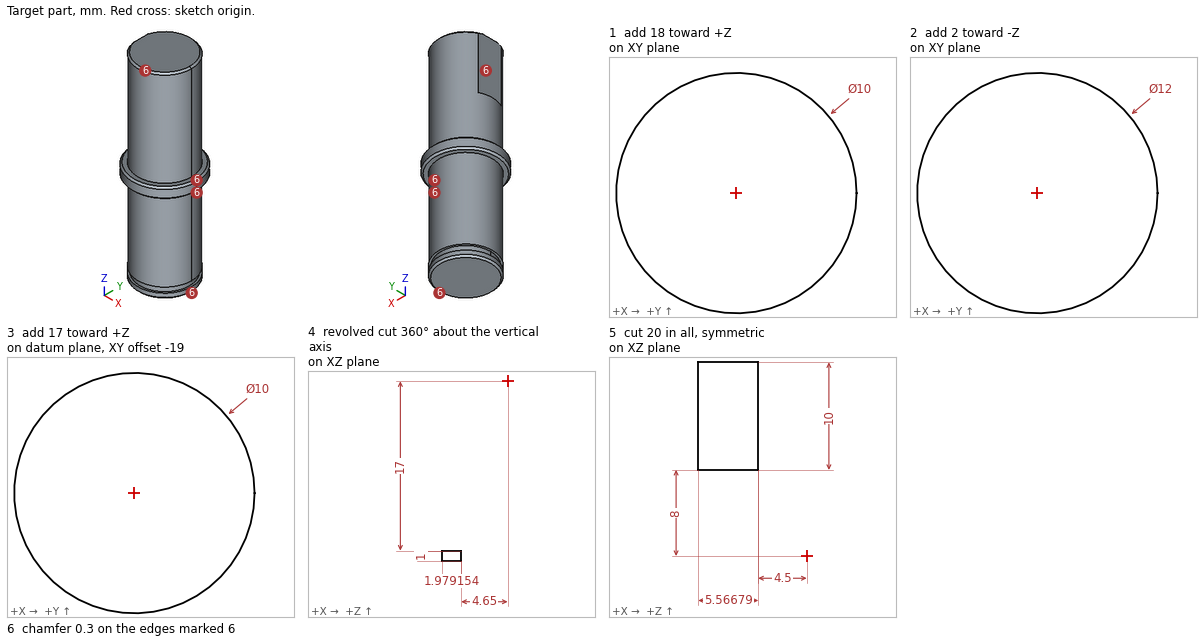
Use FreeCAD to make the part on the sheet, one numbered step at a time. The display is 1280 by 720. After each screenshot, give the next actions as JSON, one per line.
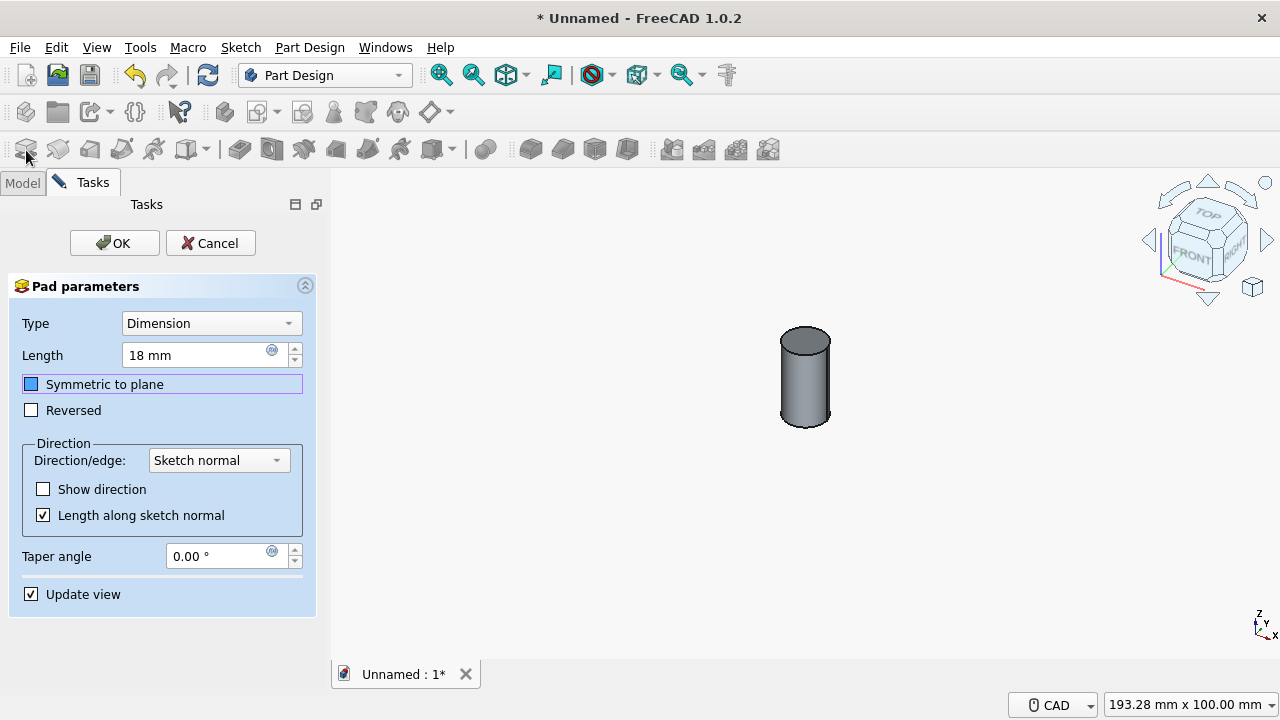
{"action": "left_click", "coordinate": [115, 243]}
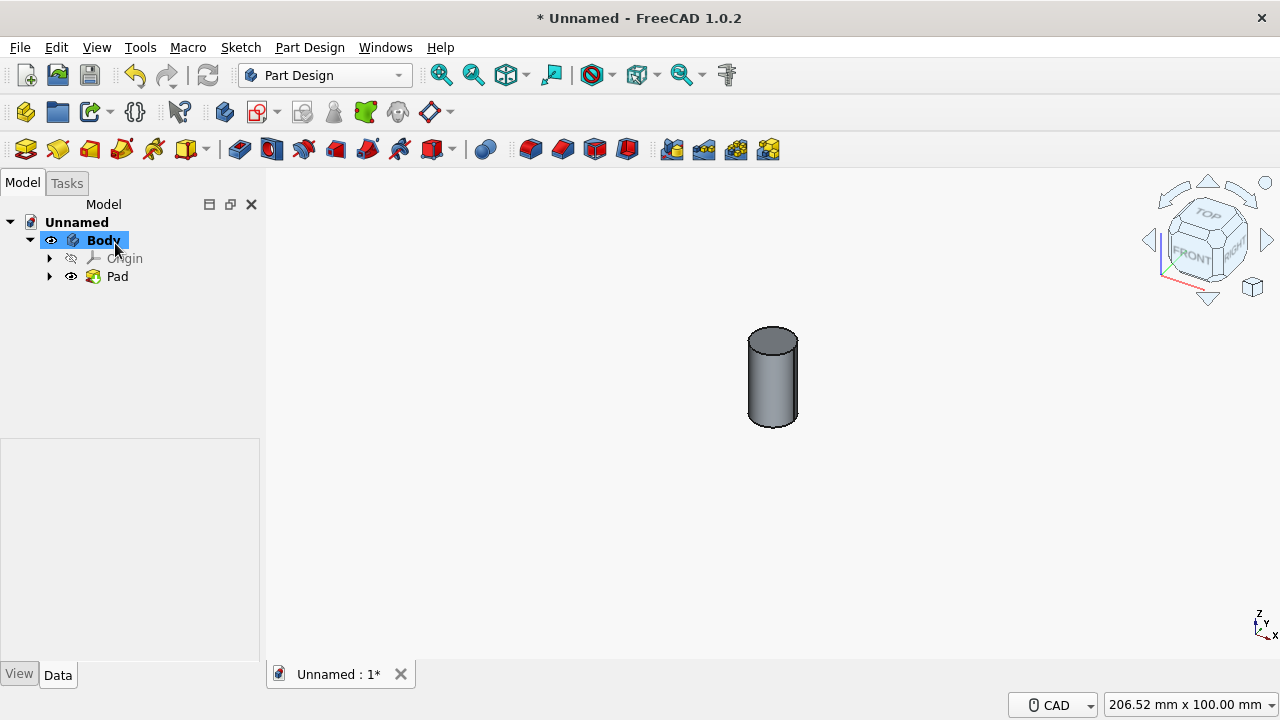
{"action": "left_click", "coordinate": [442, 76]}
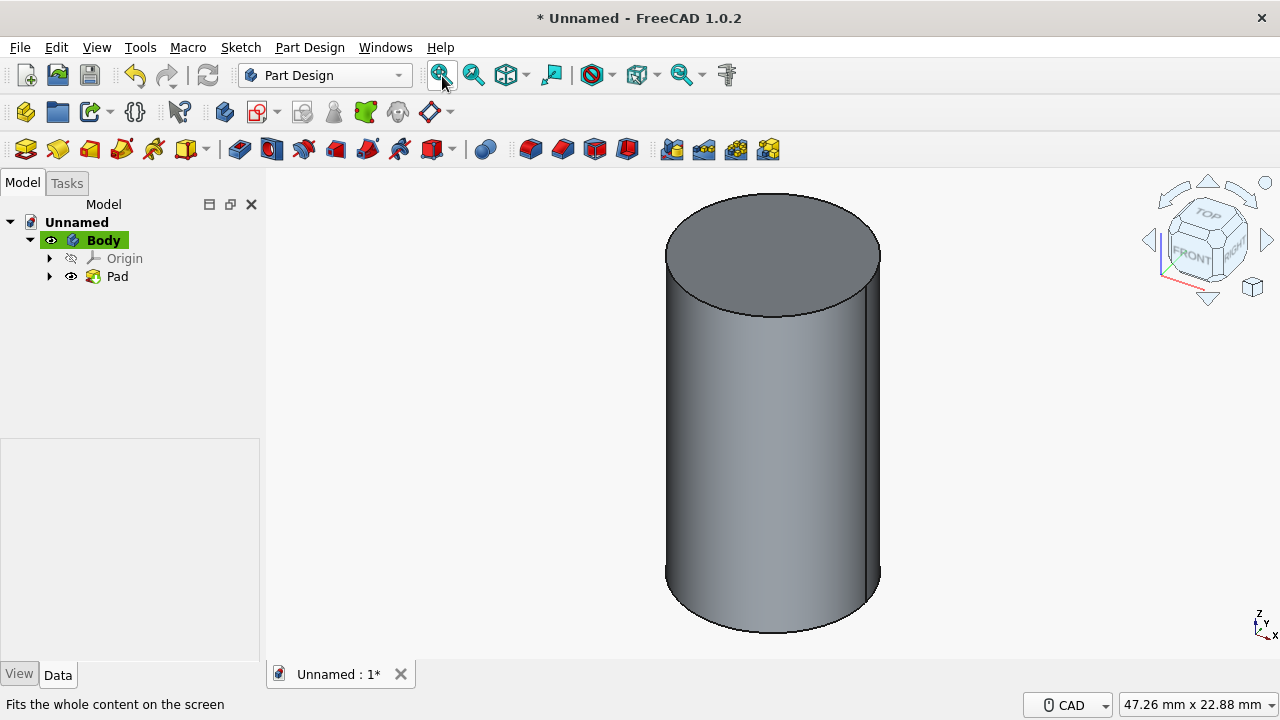
{"action": "left_click", "coordinate": [258, 112]}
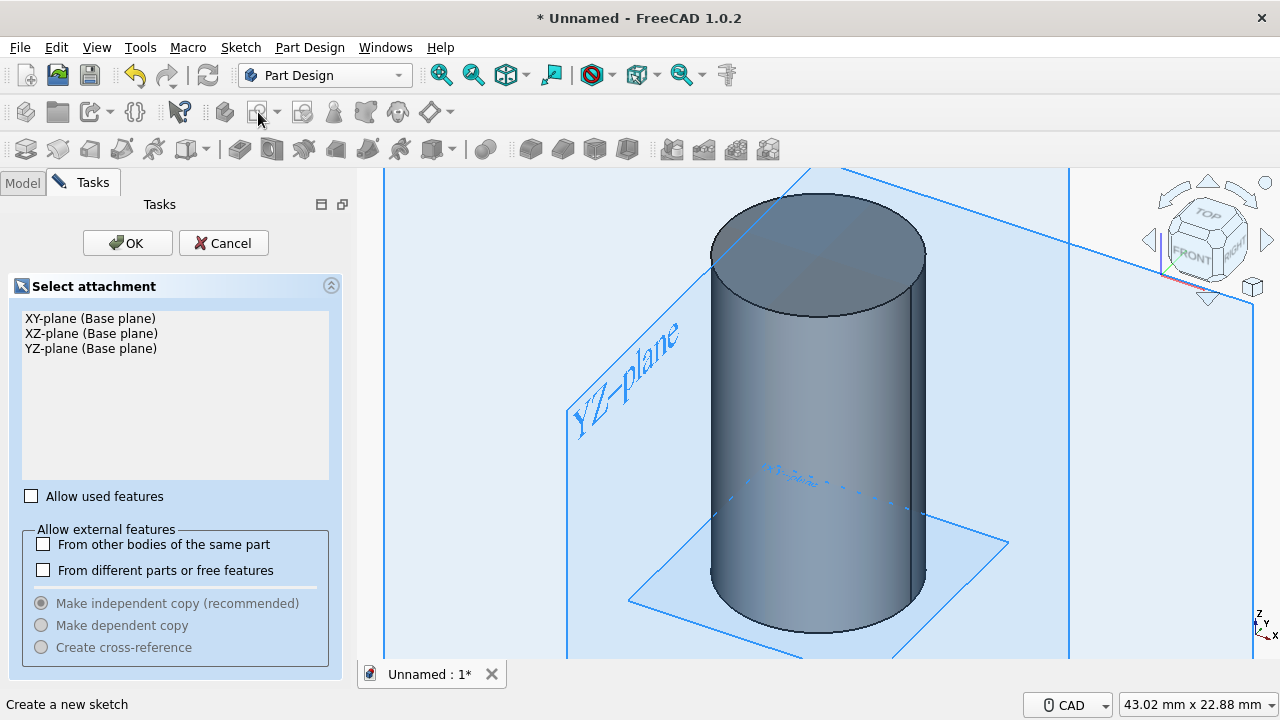
{"action": "left_click", "coordinate": [82, 318]}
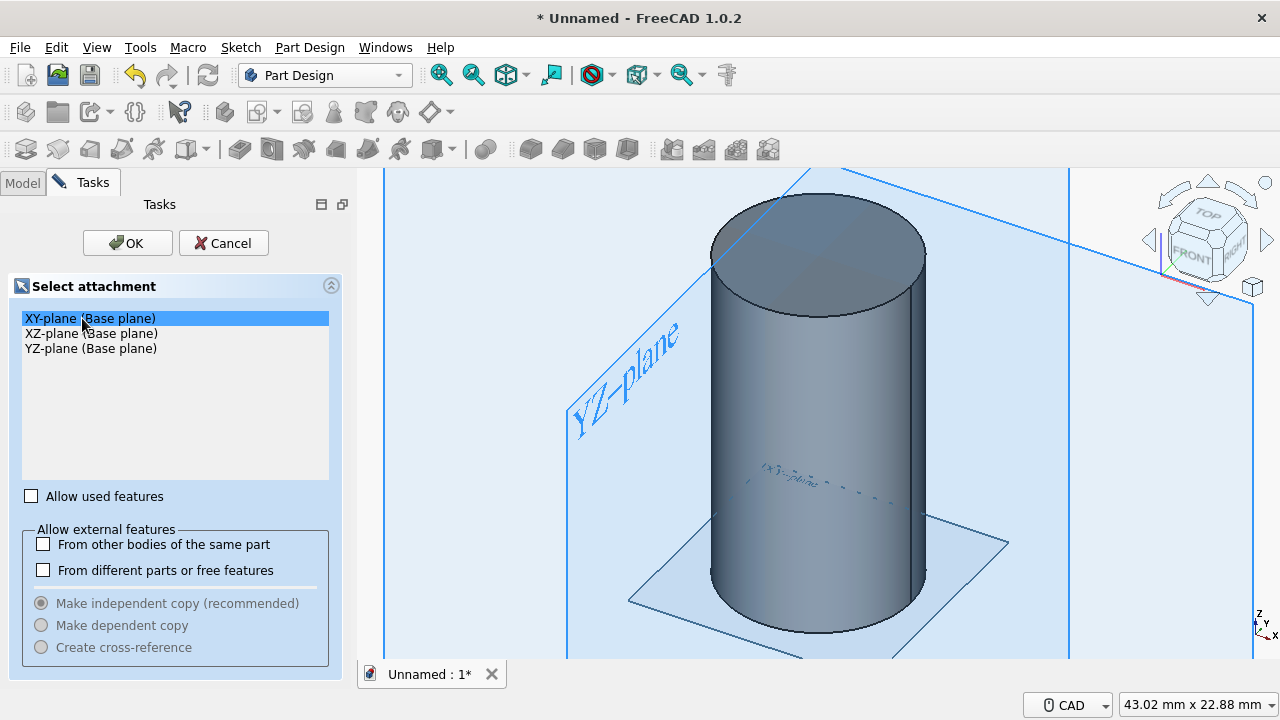
{"action": "left_click", "coordinate": [128, 243]}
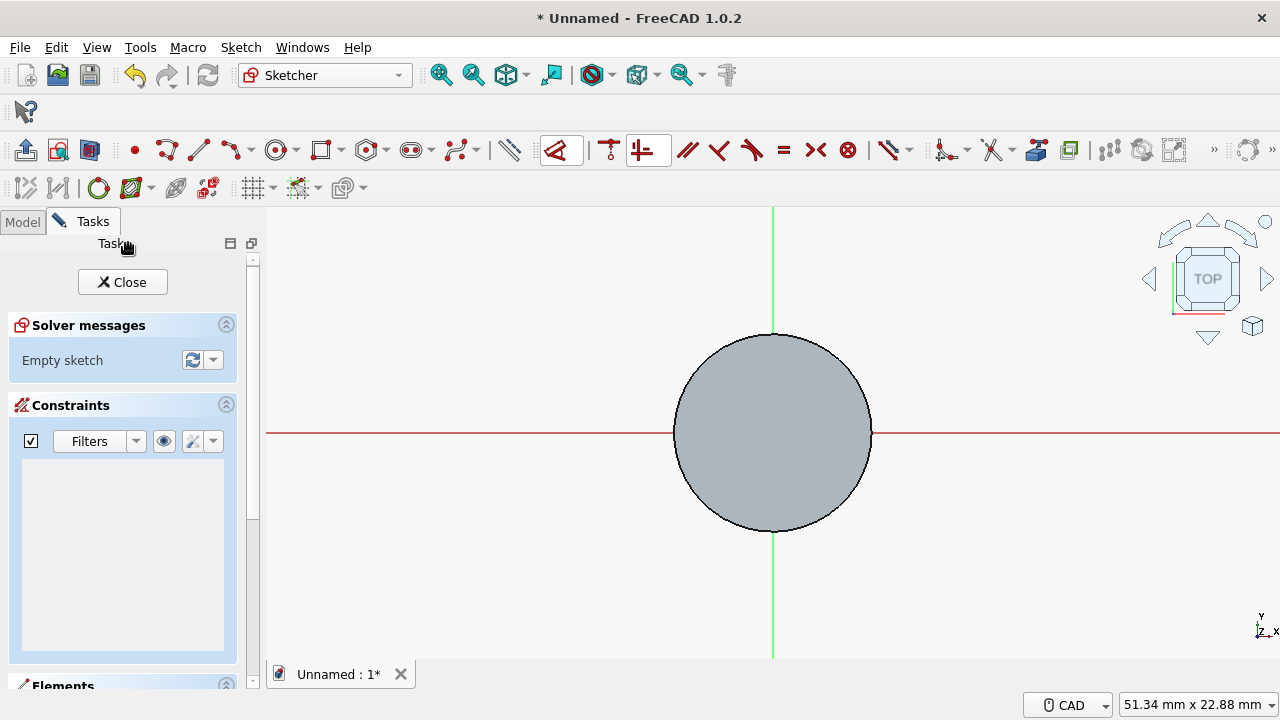
{"action": "left_click", "coordinate": [90, 150]}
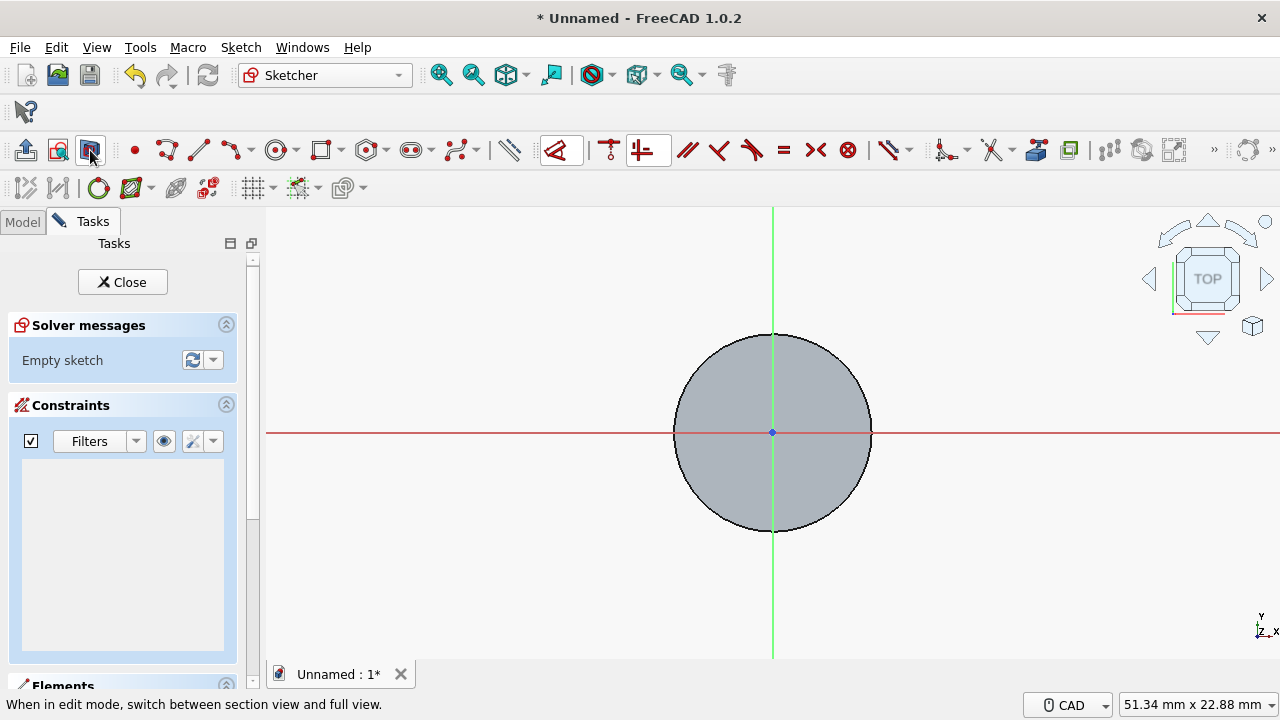
{"action": "left_click", "coordinate": [276, 150]}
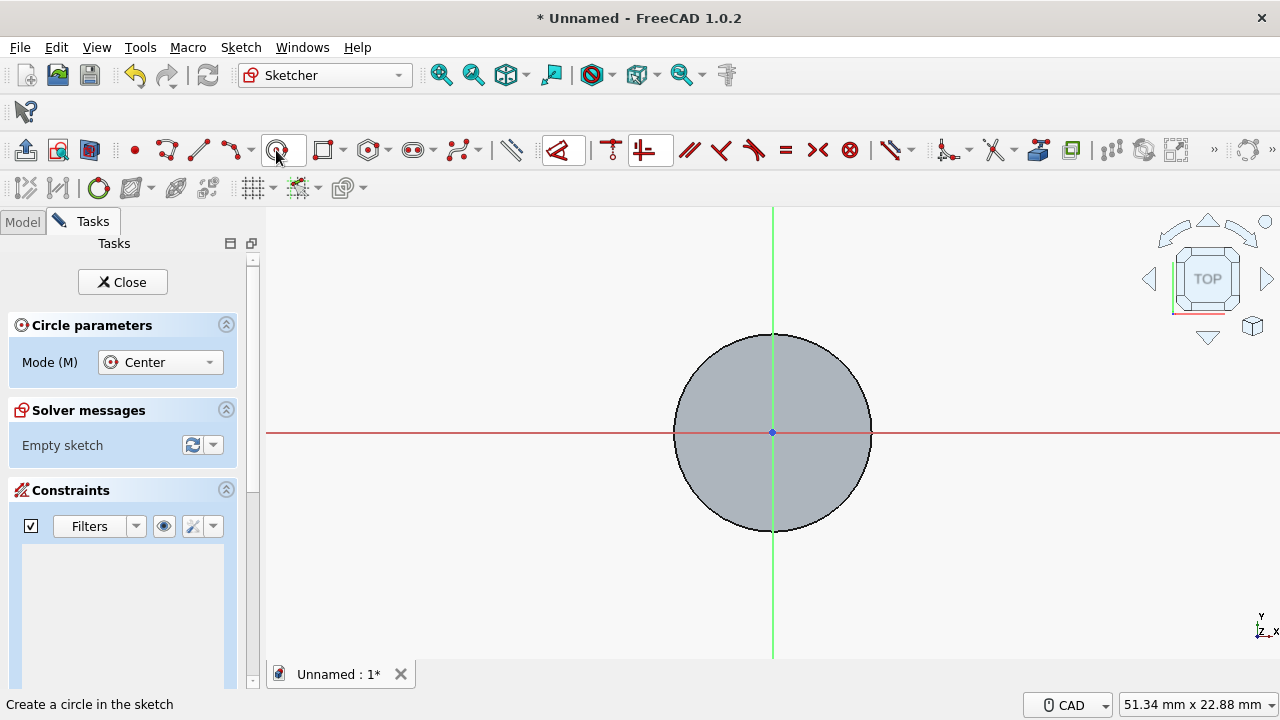
{"action": "left_click", "coordinate": [773, 433]}
{"action": "mouse_move", "coordinate": [857, 349]}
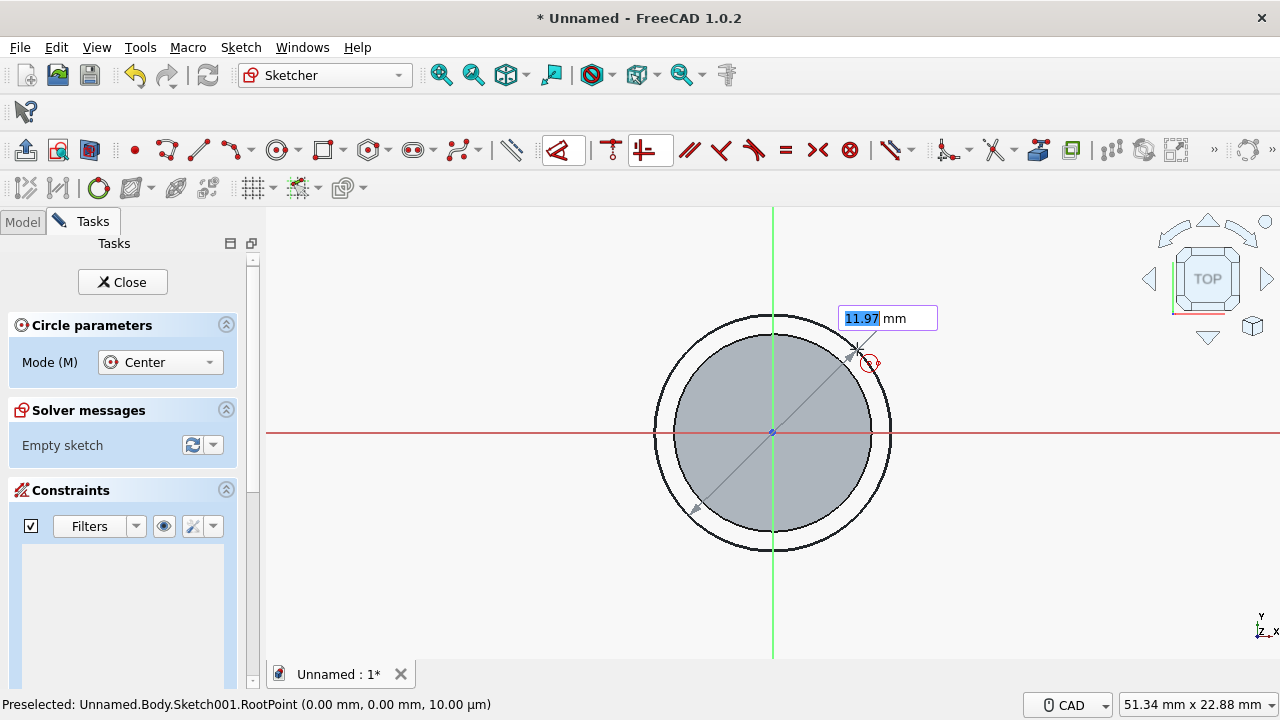
{"action": "type", "text": "12"}
{"action": "key", "text": "Return"}
{"action": "key", "text": "Escape"}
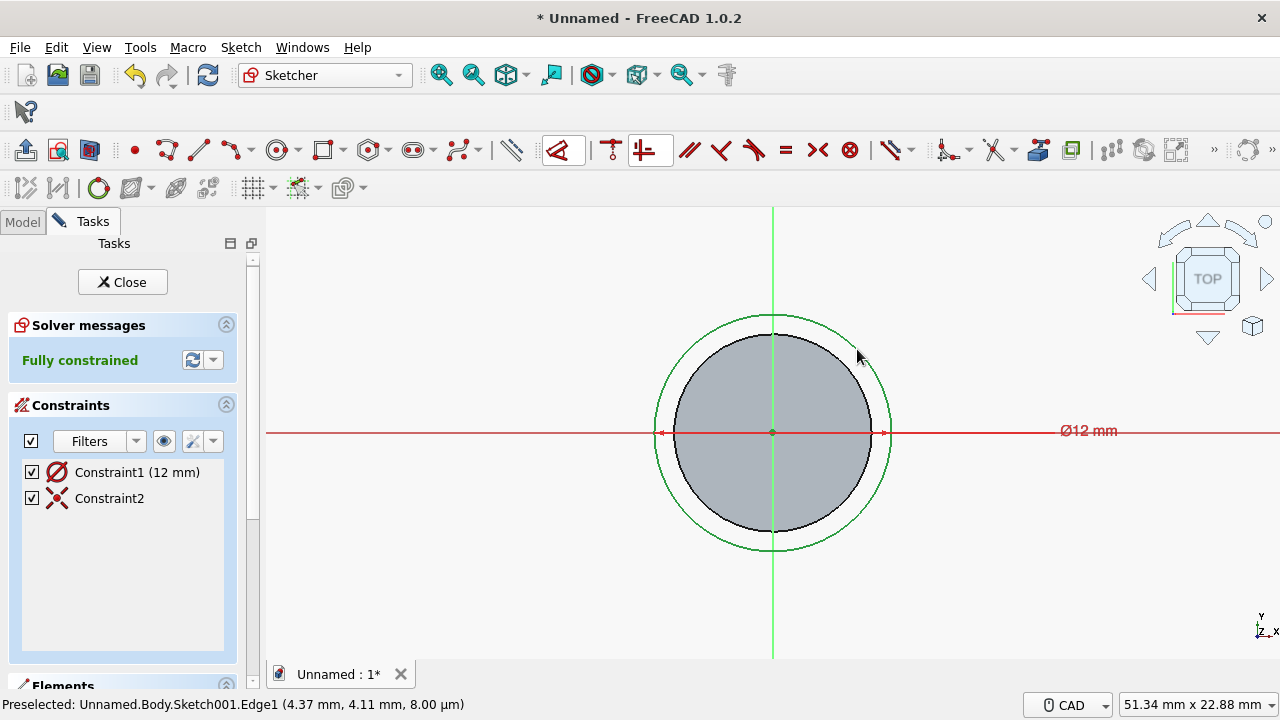
{"action": "left_click", "coordinate": [123, 282]}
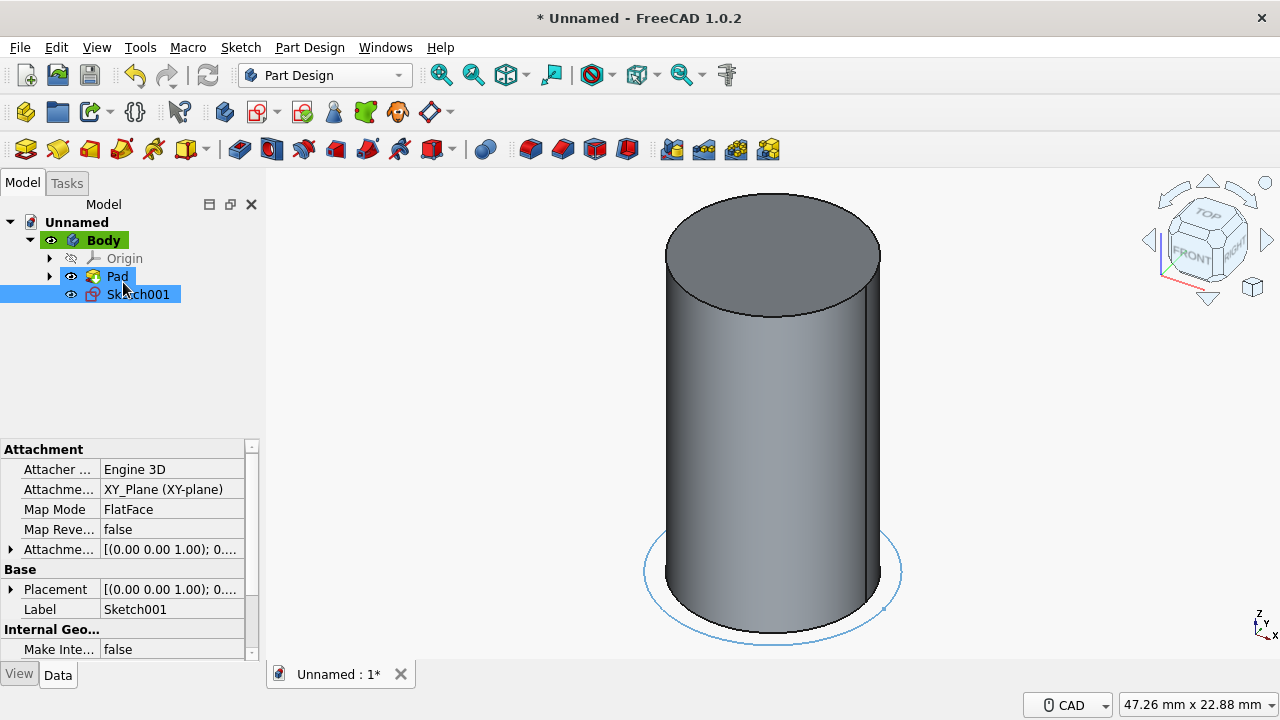
{"action": "left_click", "coordinate": [26, 150]}